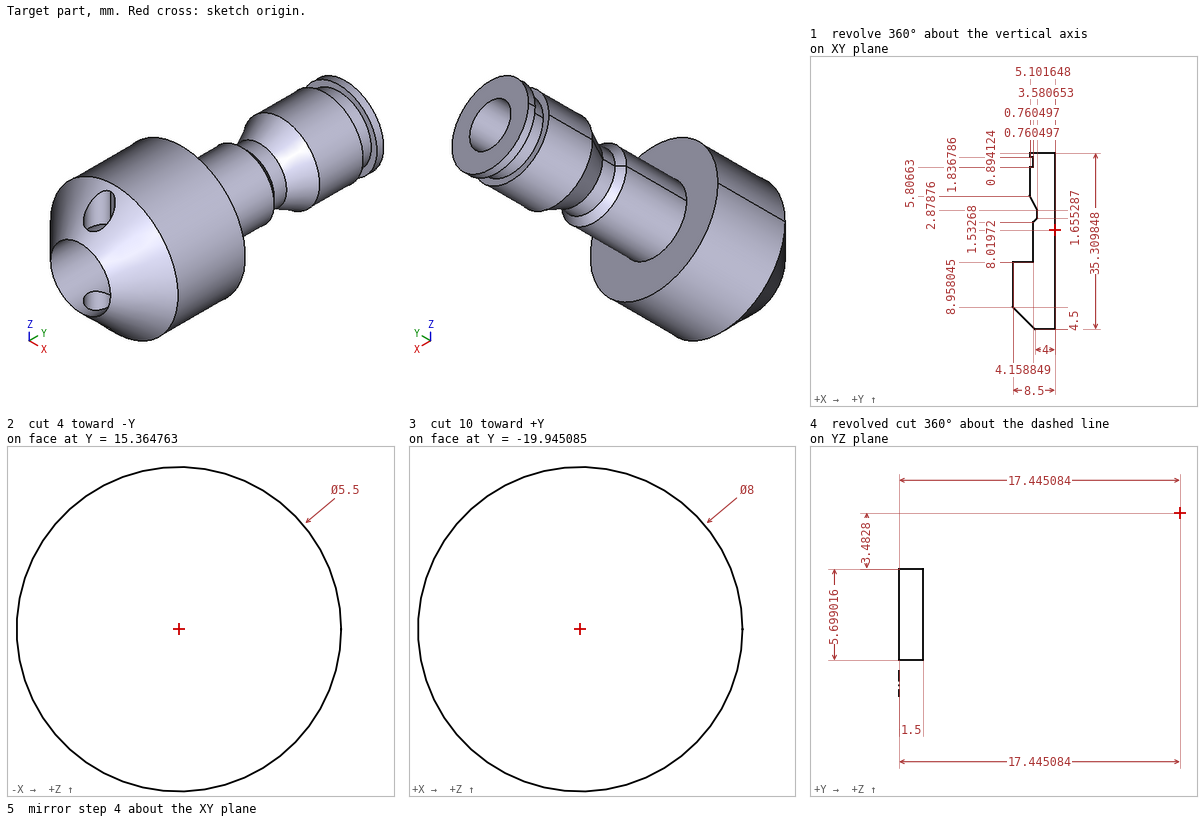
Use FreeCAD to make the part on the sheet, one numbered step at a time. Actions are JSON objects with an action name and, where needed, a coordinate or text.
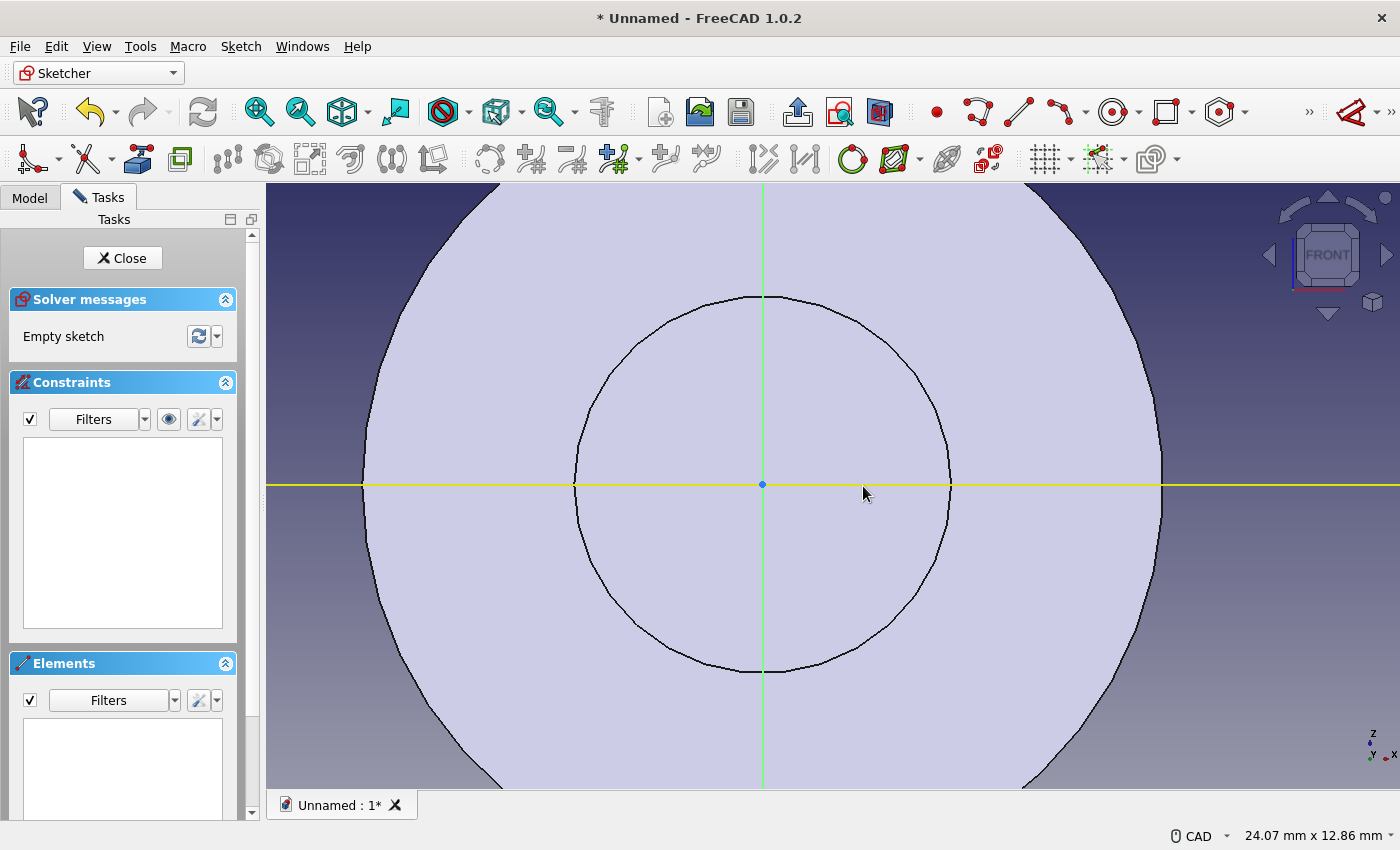
{"action": "left_click", "coordinate": [1112, 112]}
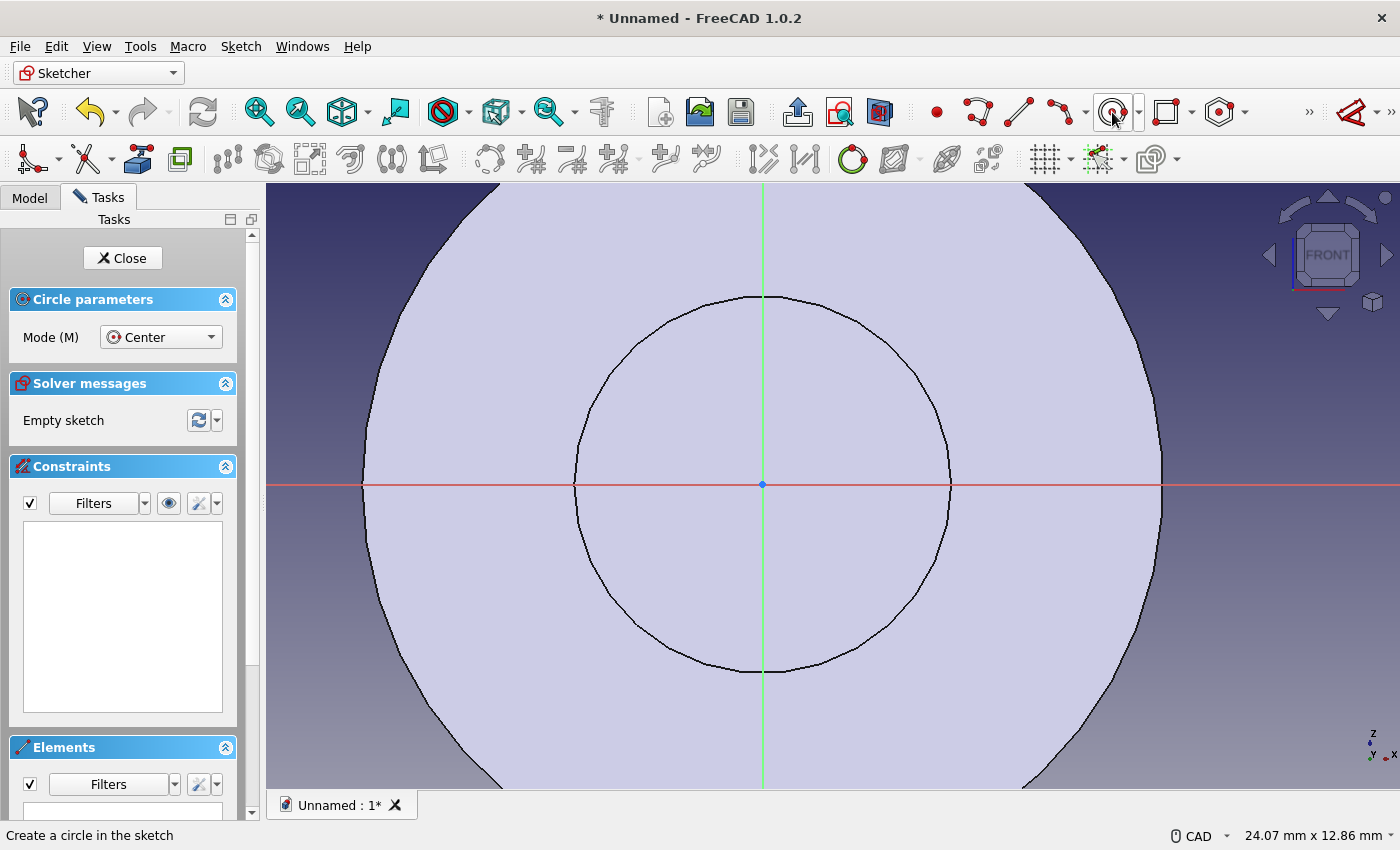
{"action": "left_click", "coordinate": [763, 485]}
{"action": "left_click", "coordinate": [896, 352]}
{"action": "key", "text": "Escape"}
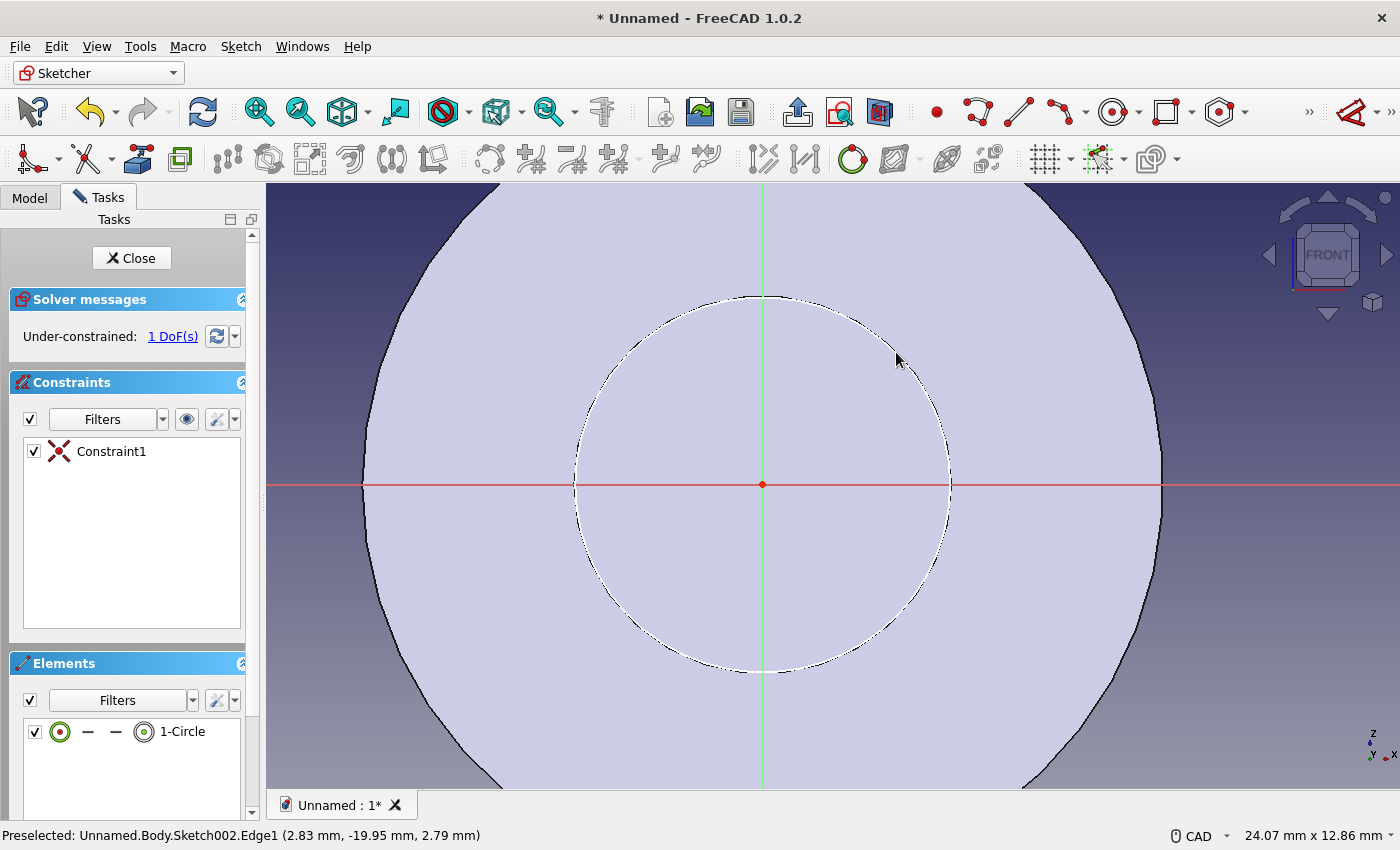
{"action": "left_click", "coordinate": [1350, 112]}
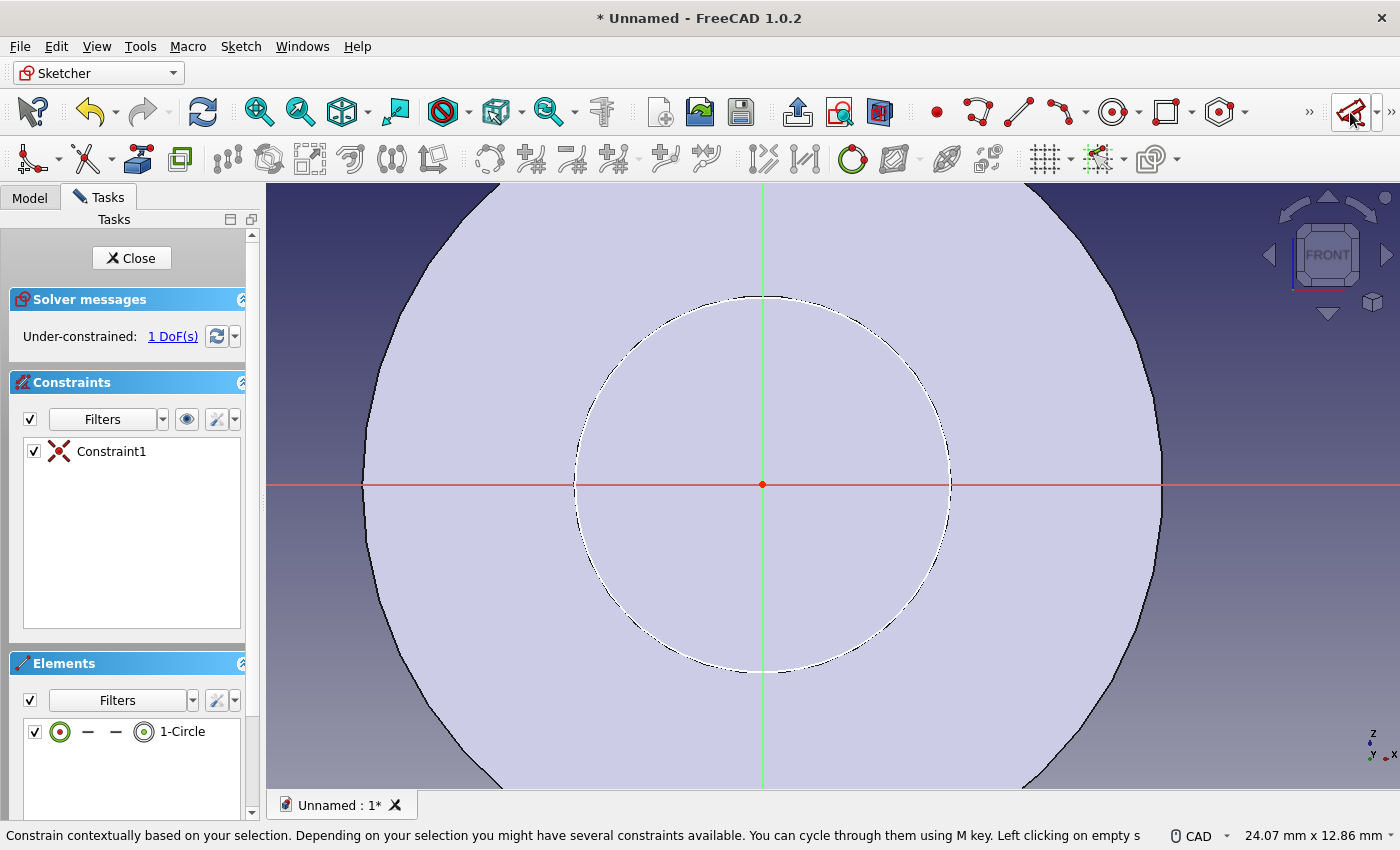
{"action": "left_click", "coordinate": [895, 352]}
{"action": "left_click", "coordinate": [918, 329]}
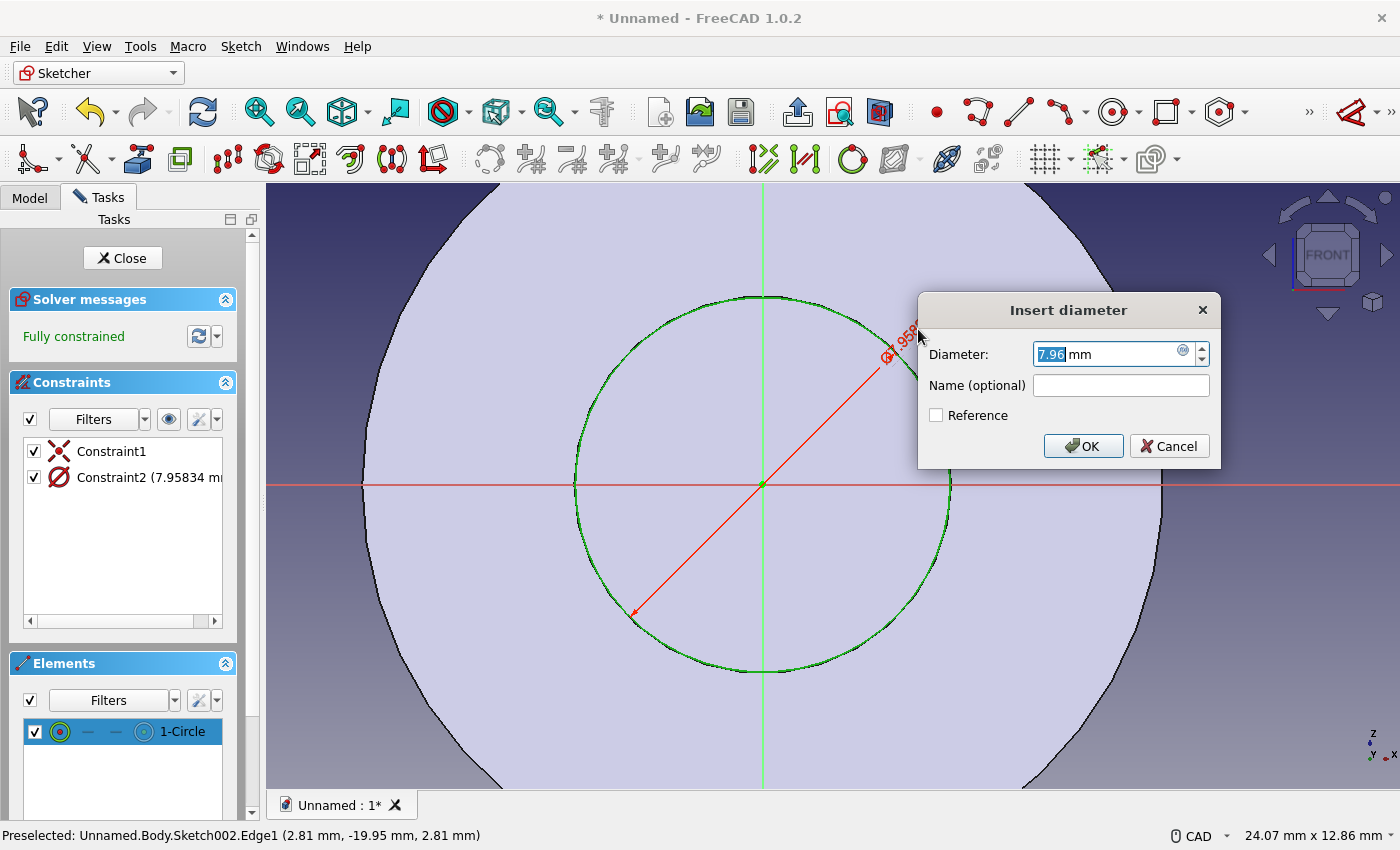
{"action": "type", "text": "8"}
{"action": "key", "text": "Return"}
{"action": "key", "text": "Escape"}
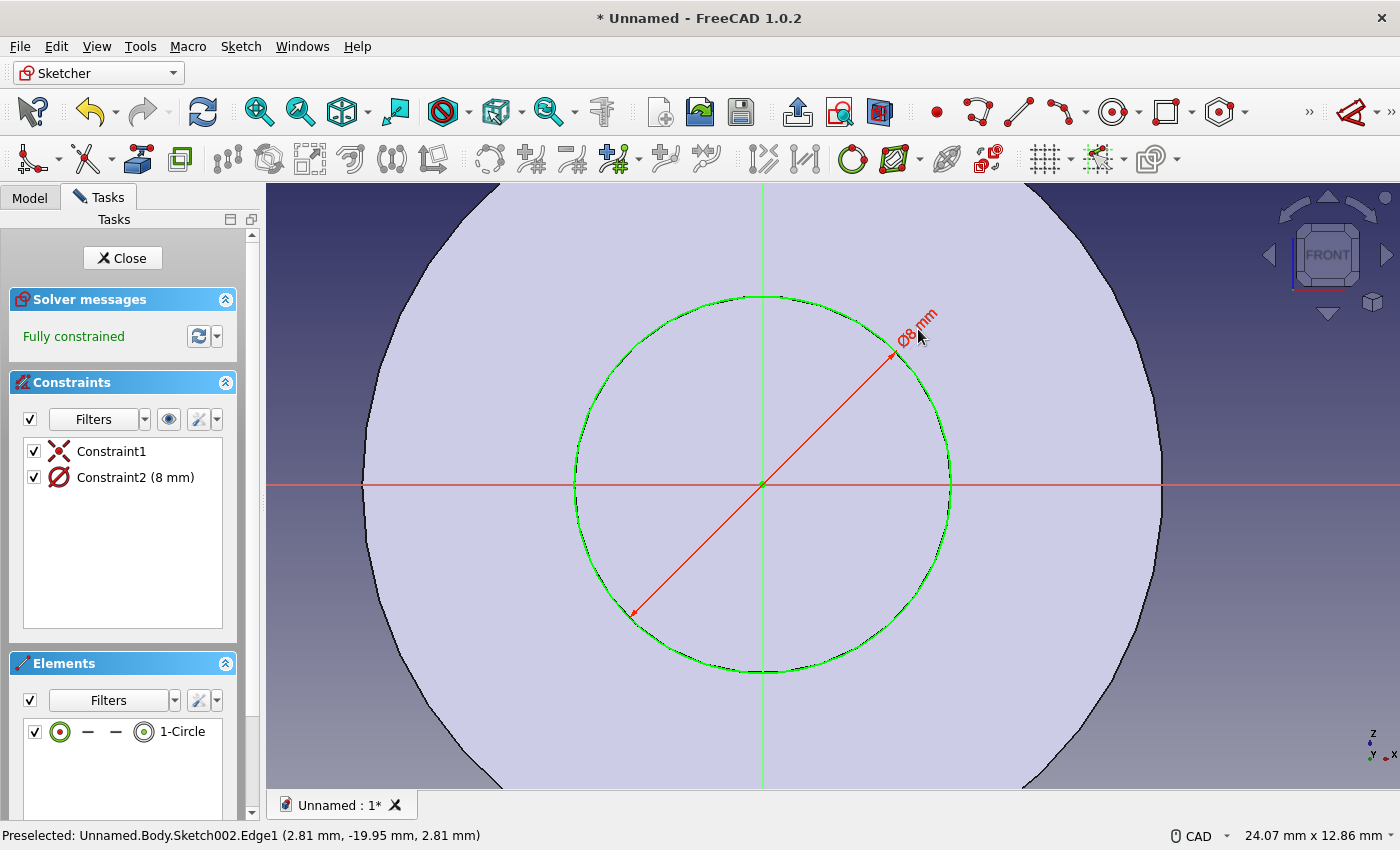
{"action": "left_click", "coordinate": [123, 258]}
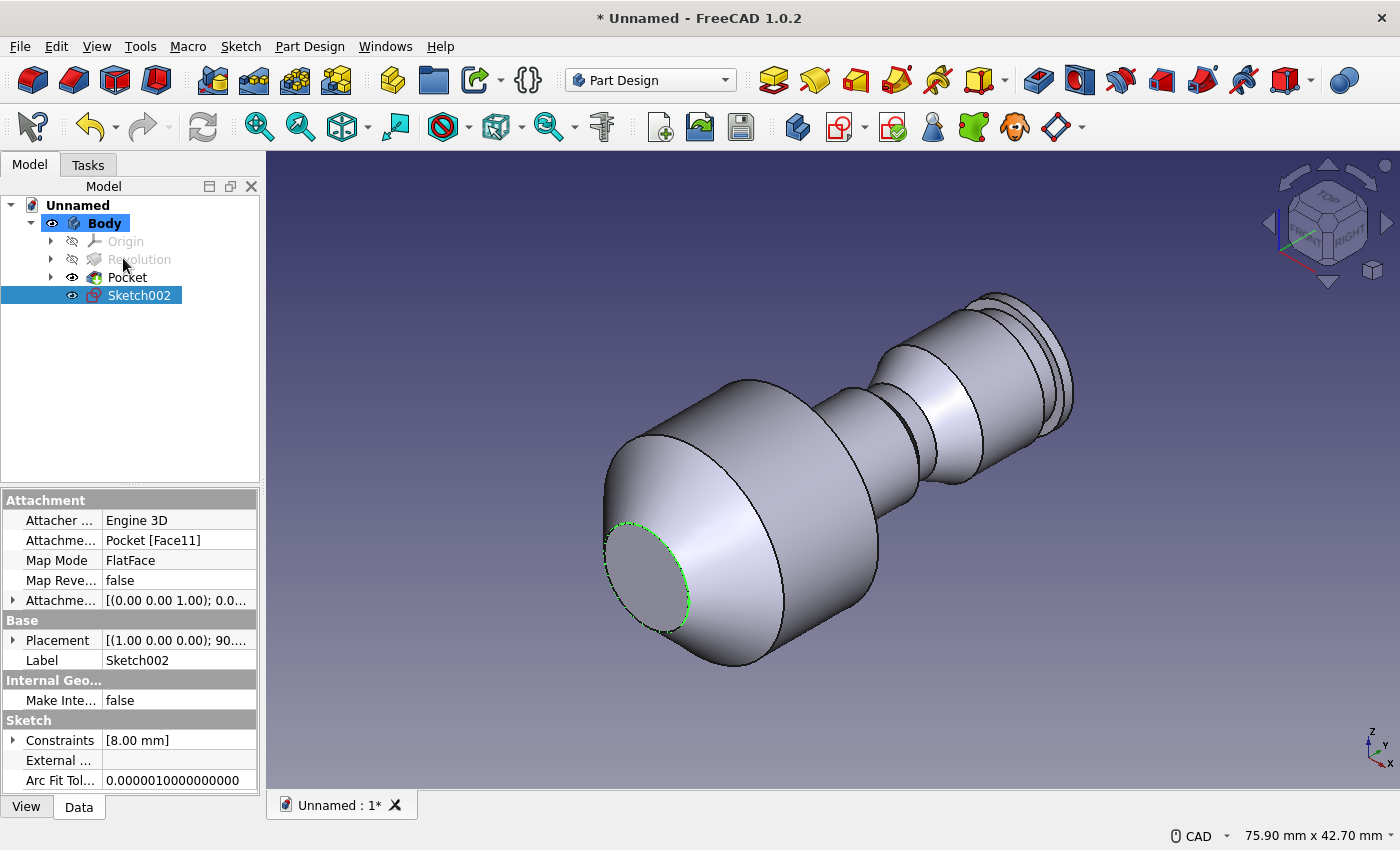
{"action": "left_click", "coordinate": [1039, 80]}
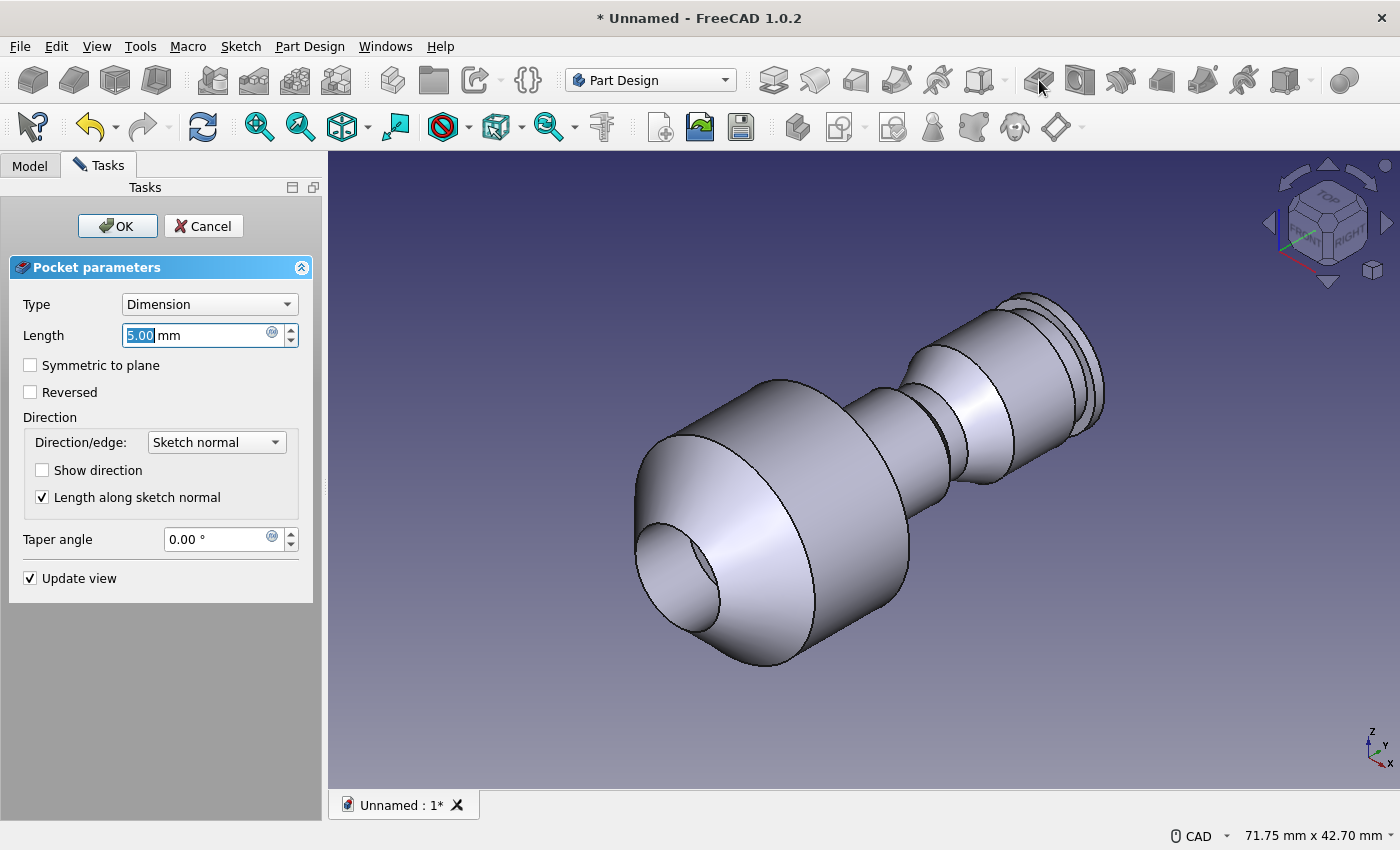
{"action": "type", "text": "10"}
{"action": "key", "text": "Tab"}